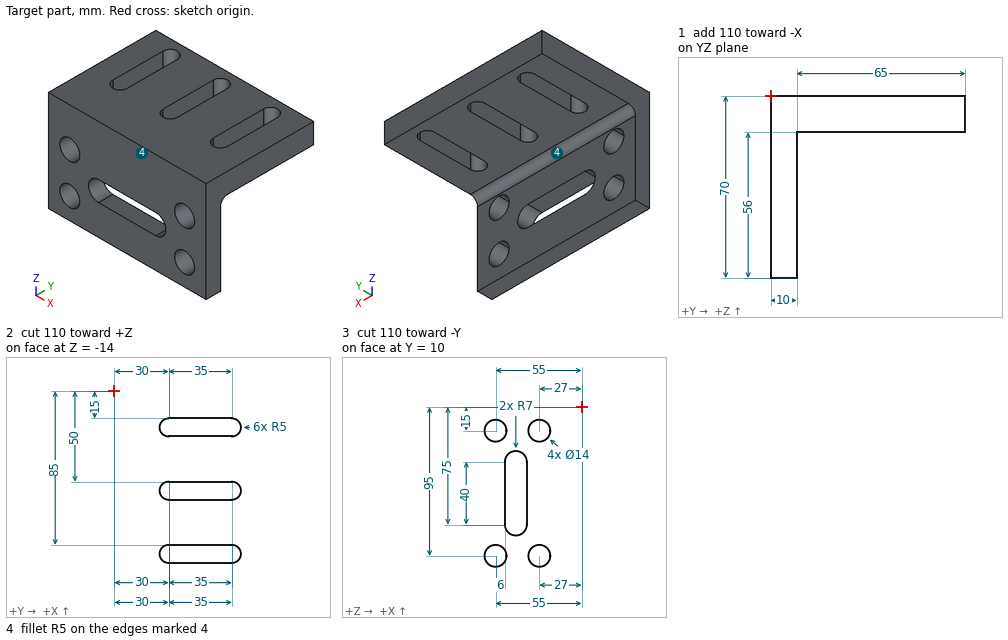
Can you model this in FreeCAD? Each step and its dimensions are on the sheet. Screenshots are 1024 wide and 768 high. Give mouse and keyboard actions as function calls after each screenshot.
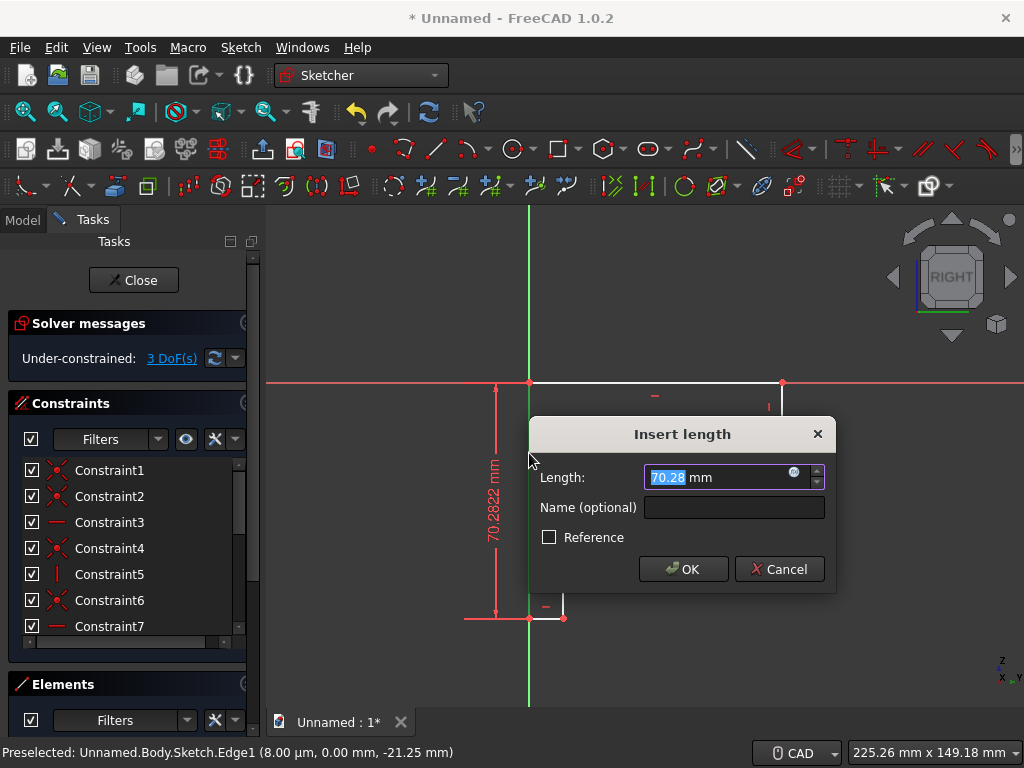
text(70)
key(Return)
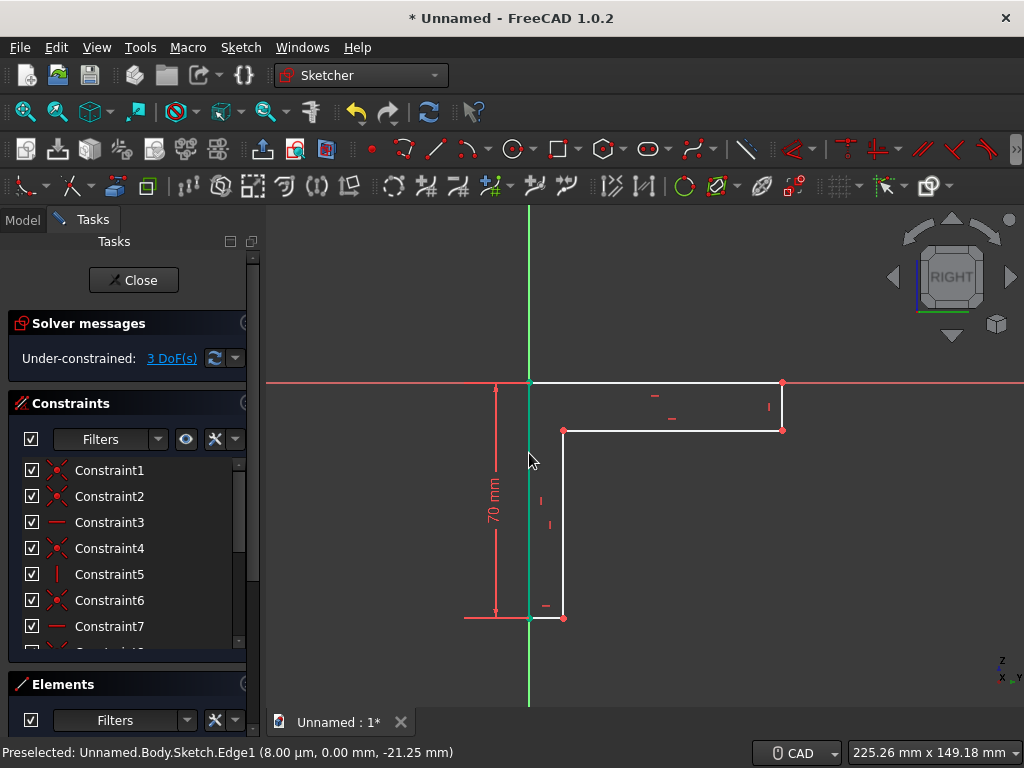
scroll(539, 618, up, 2)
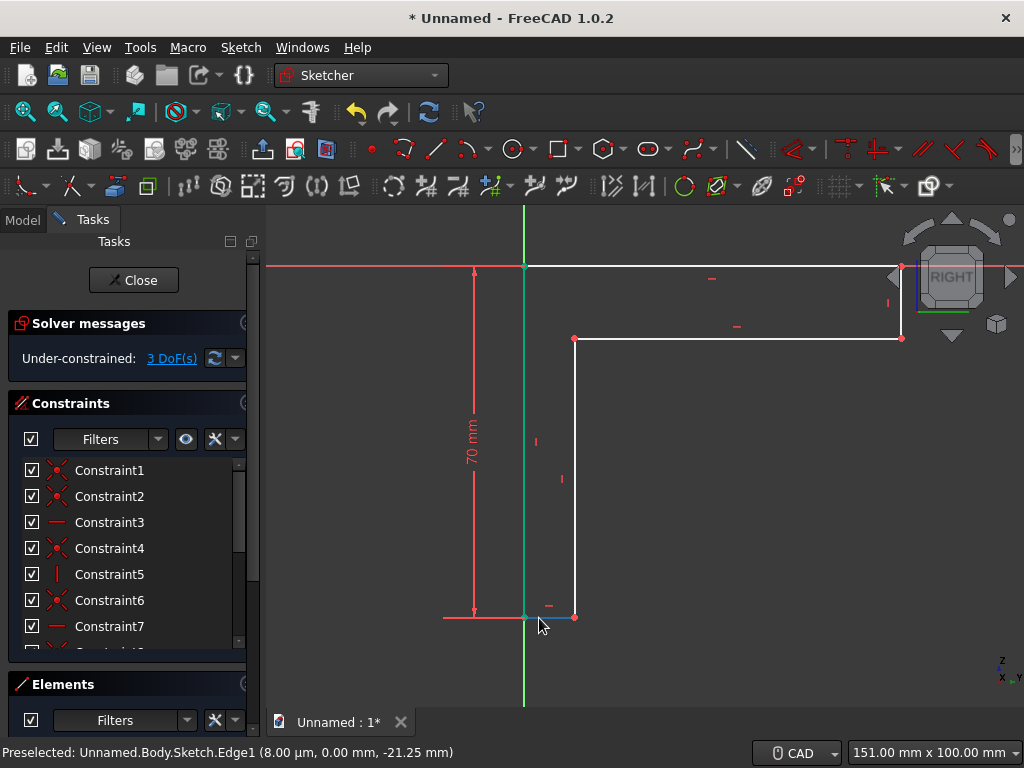
click(539, 618)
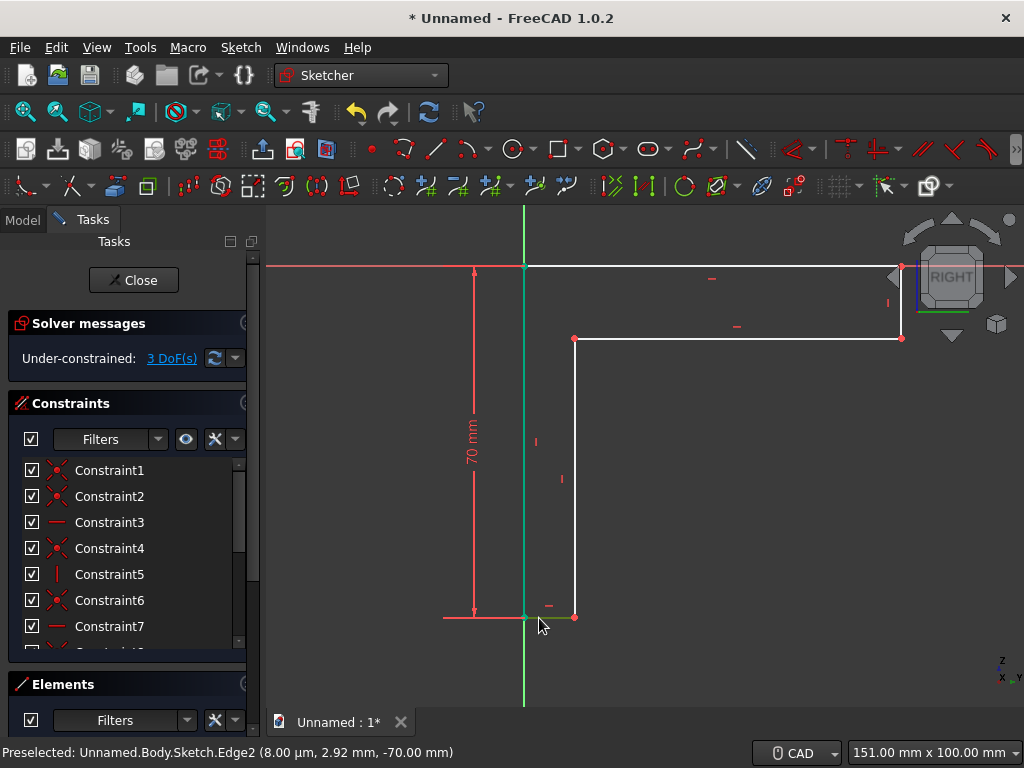
click(814, 150)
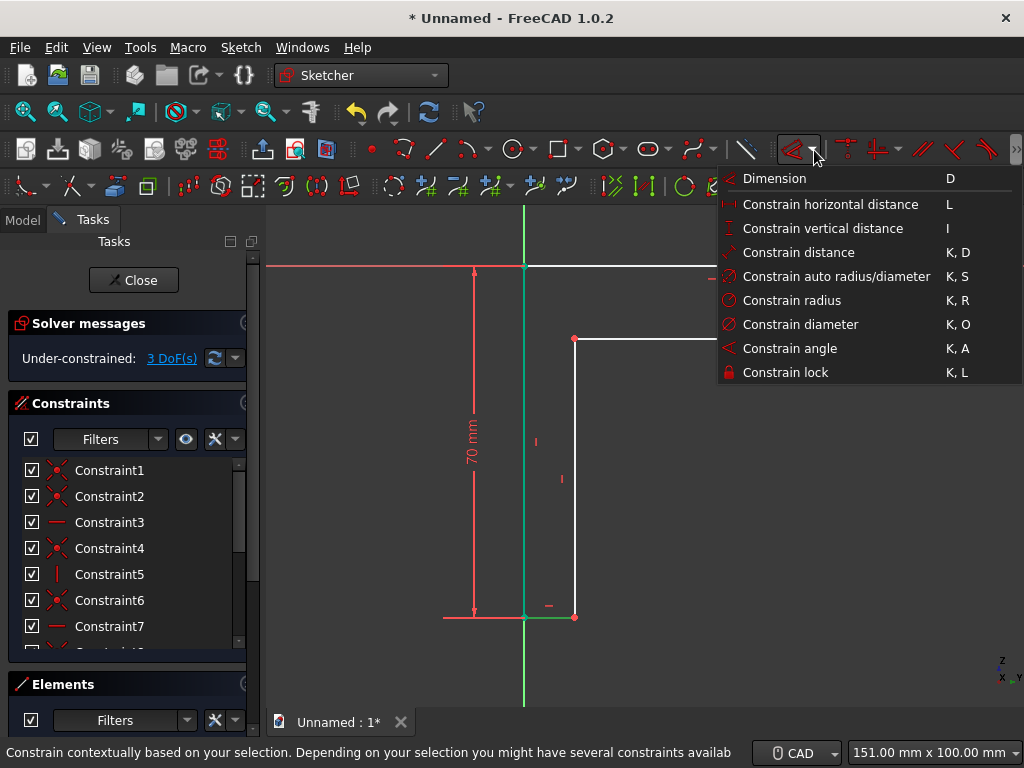
click(870, 204)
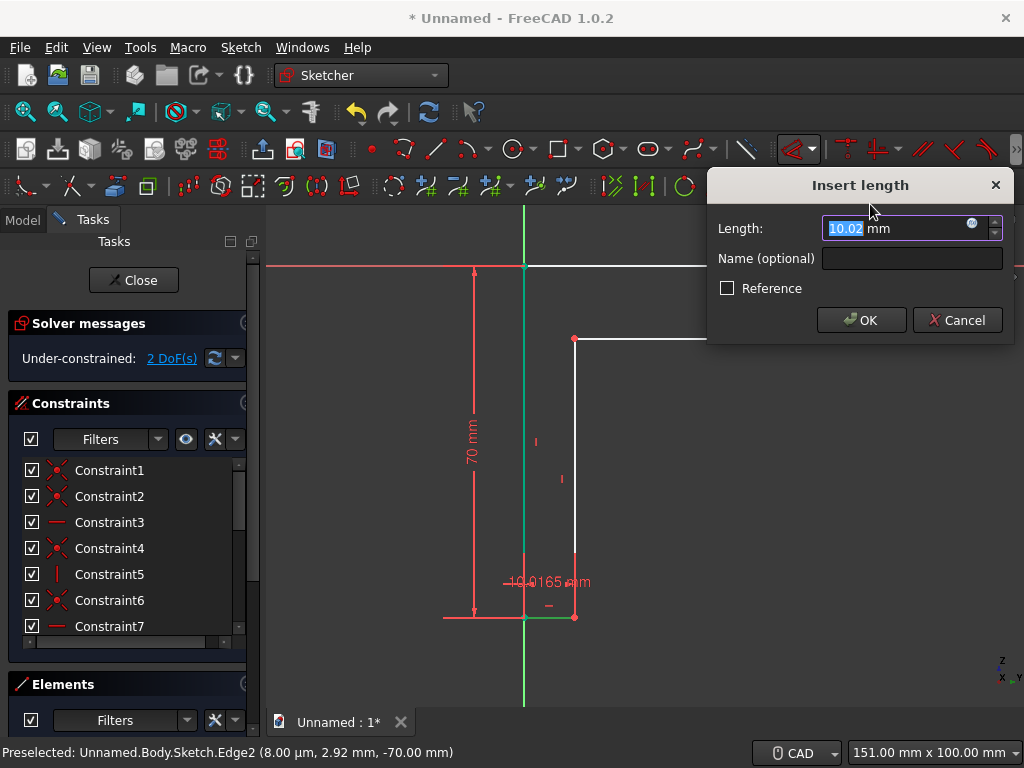
text(10)
key(Return)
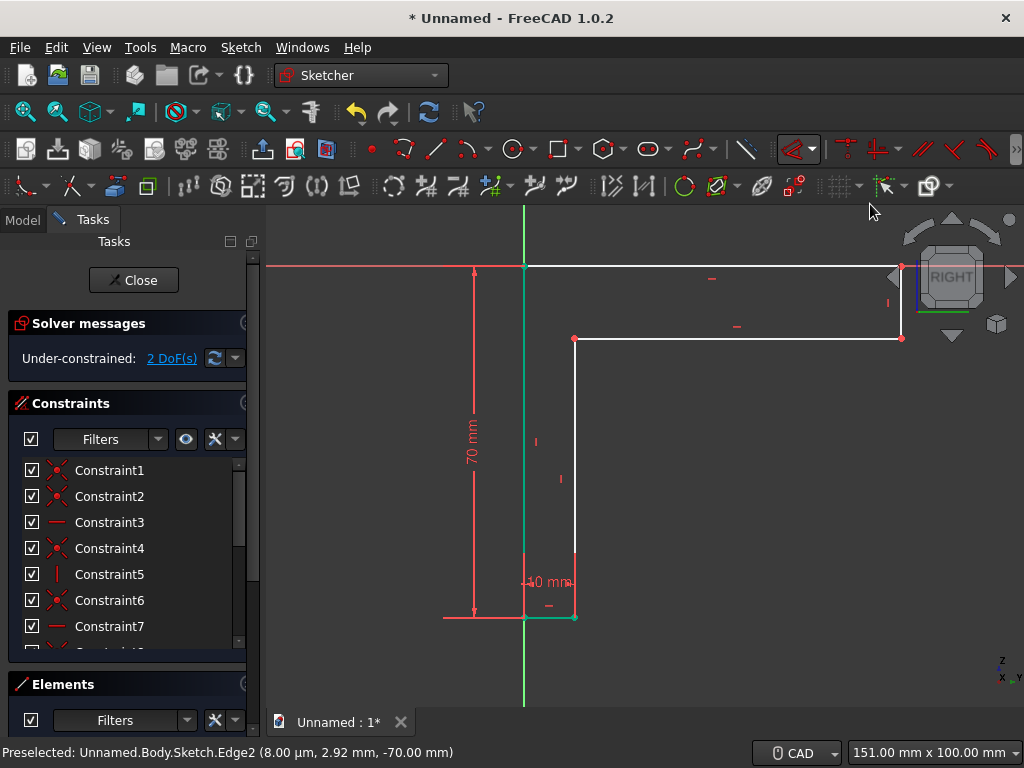
click(575, 534)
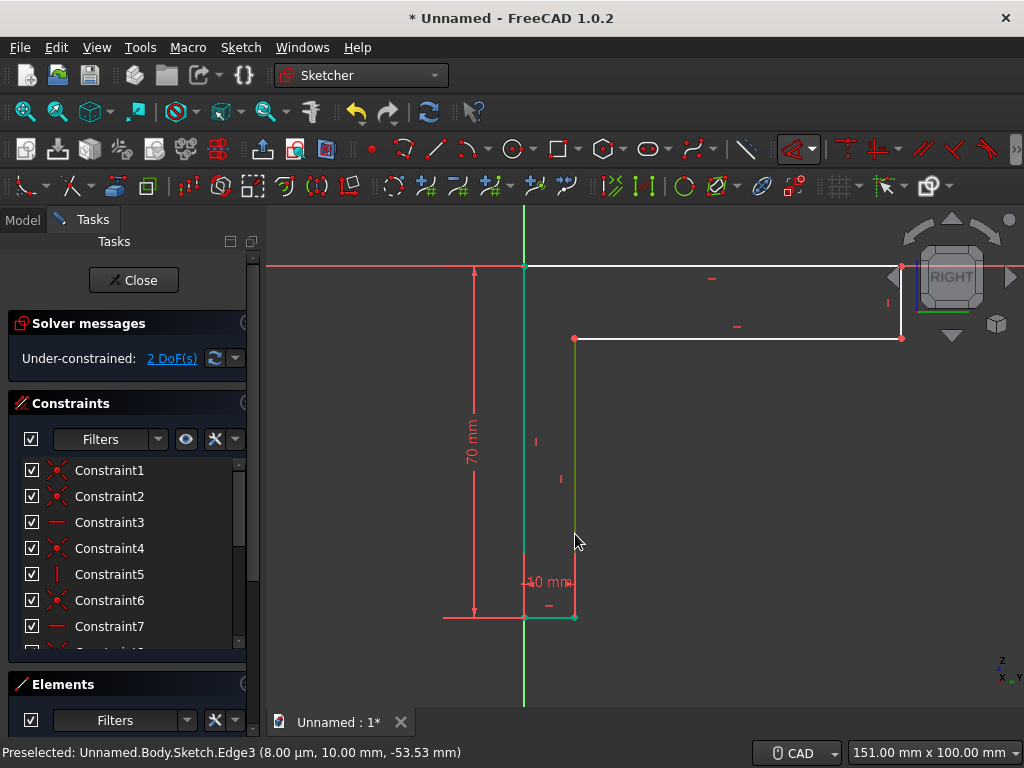
key(i)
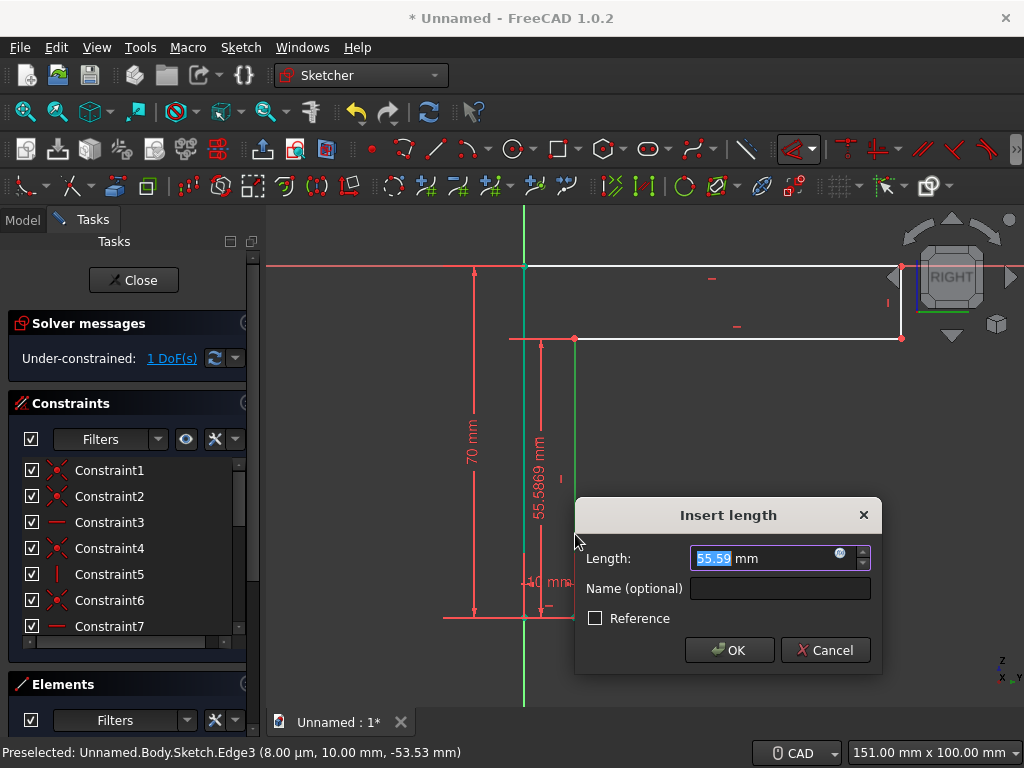
text(56)
key(Return)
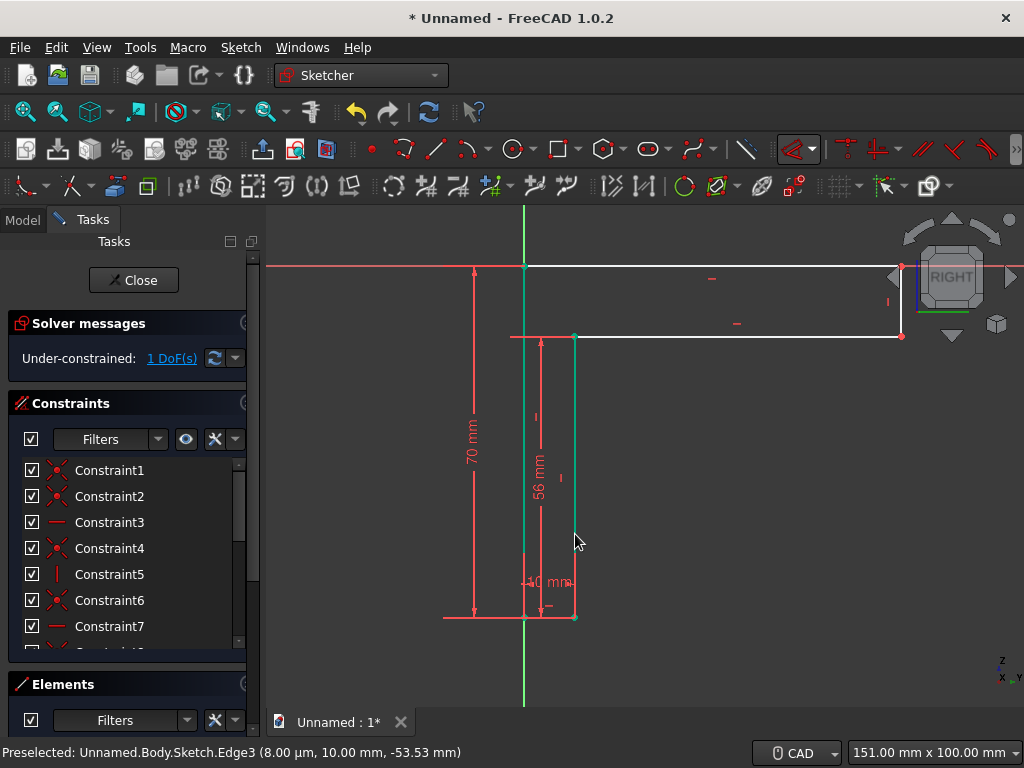
click(673, 337)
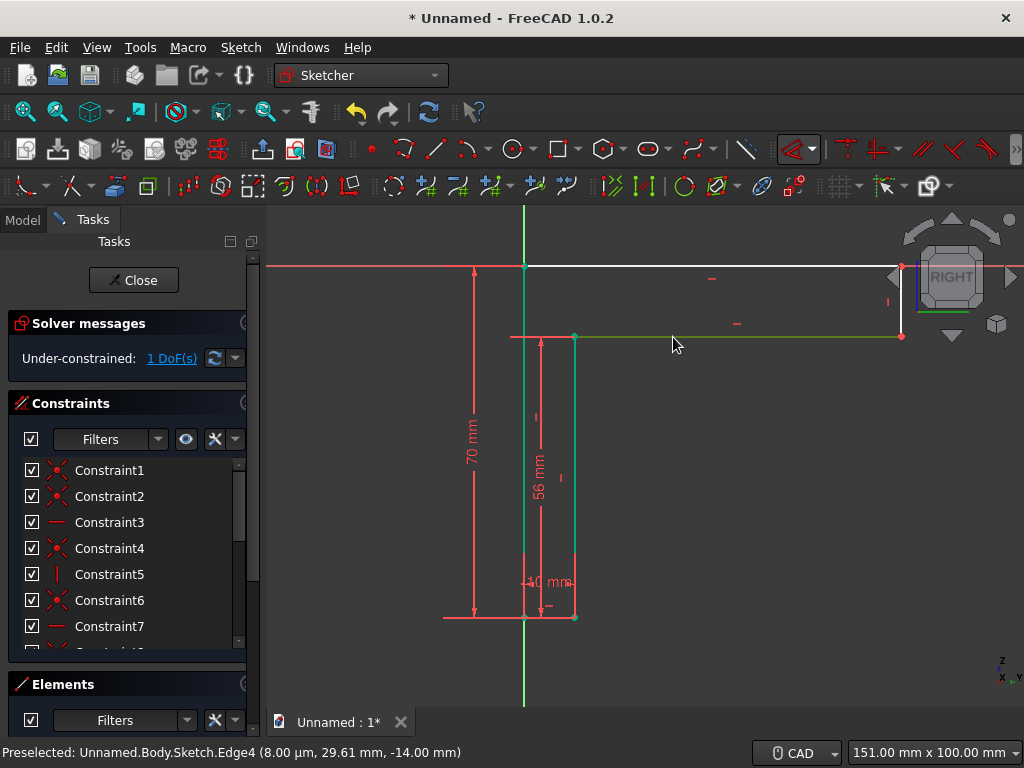
key(l)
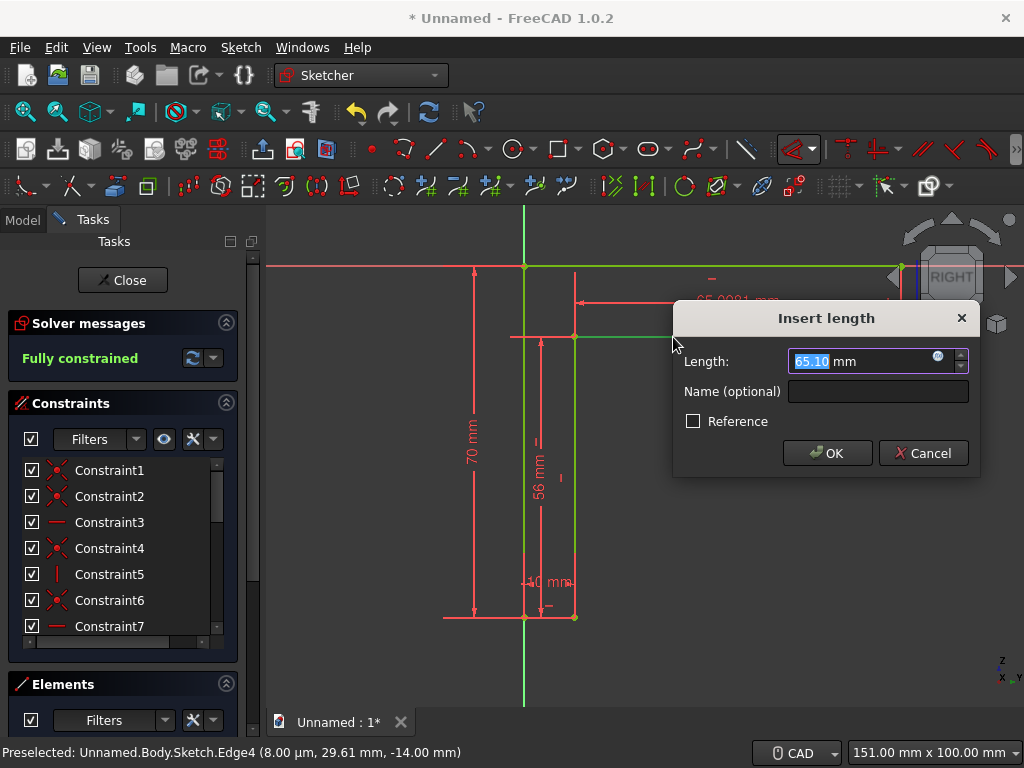
text(65)
key(Return)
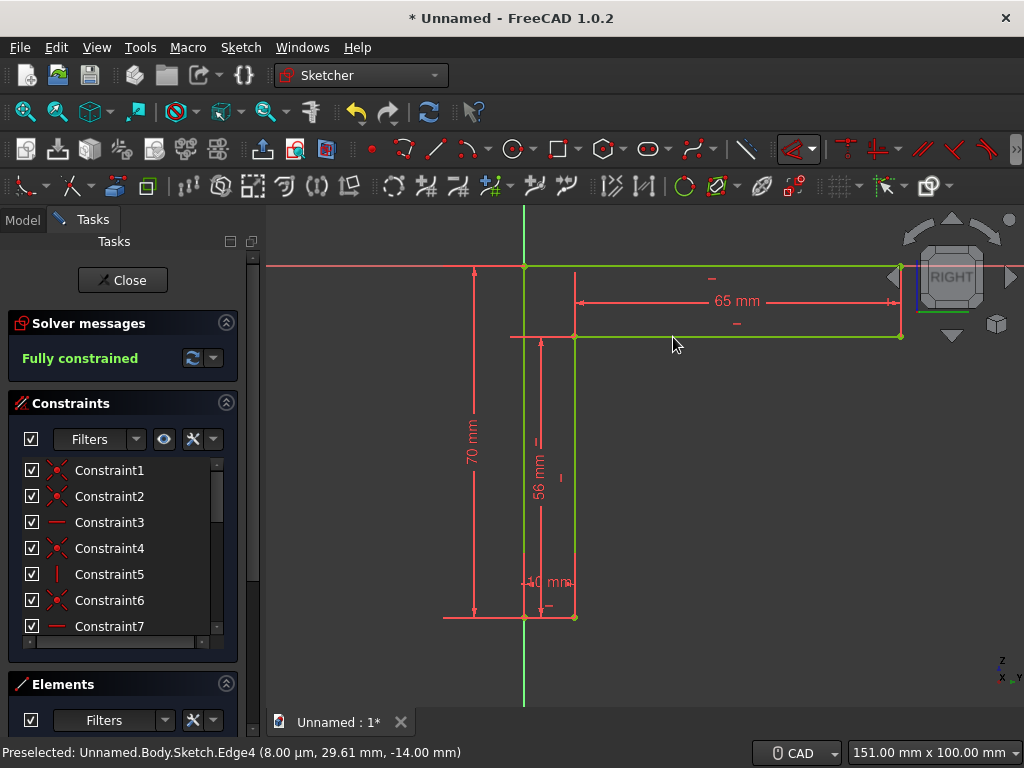
click(123, 280)